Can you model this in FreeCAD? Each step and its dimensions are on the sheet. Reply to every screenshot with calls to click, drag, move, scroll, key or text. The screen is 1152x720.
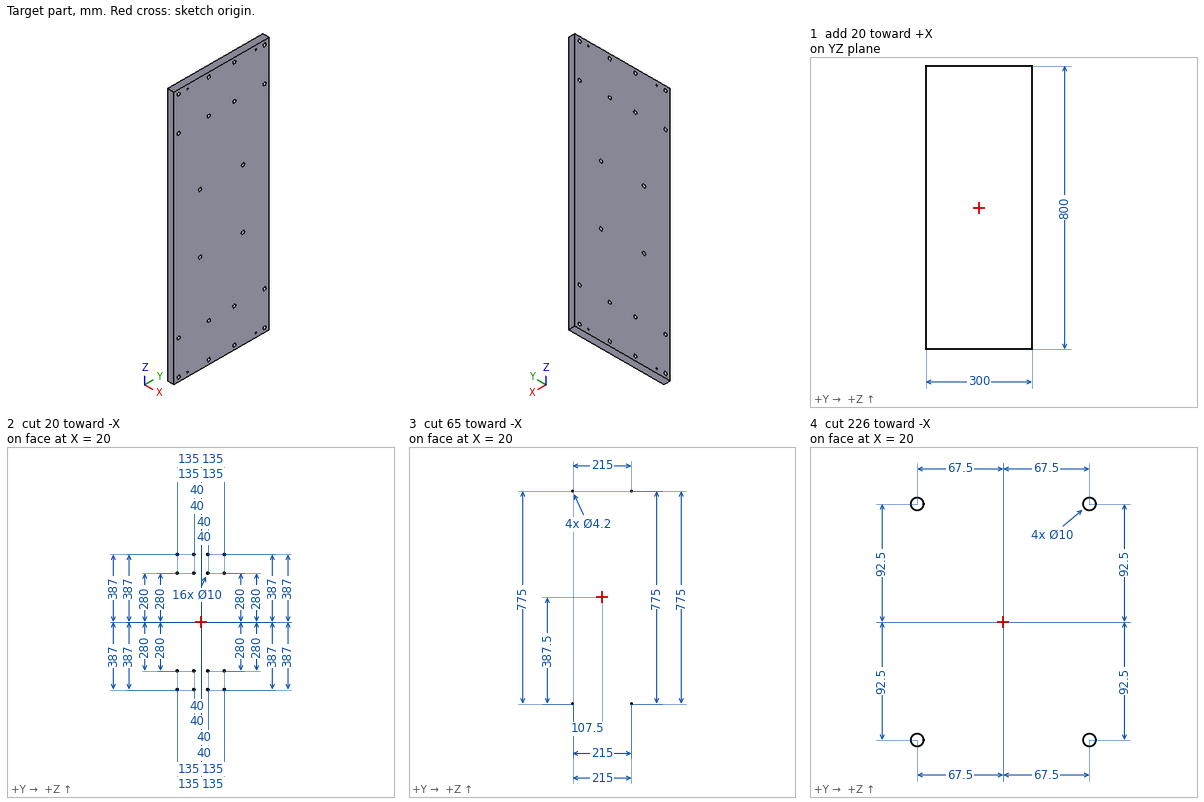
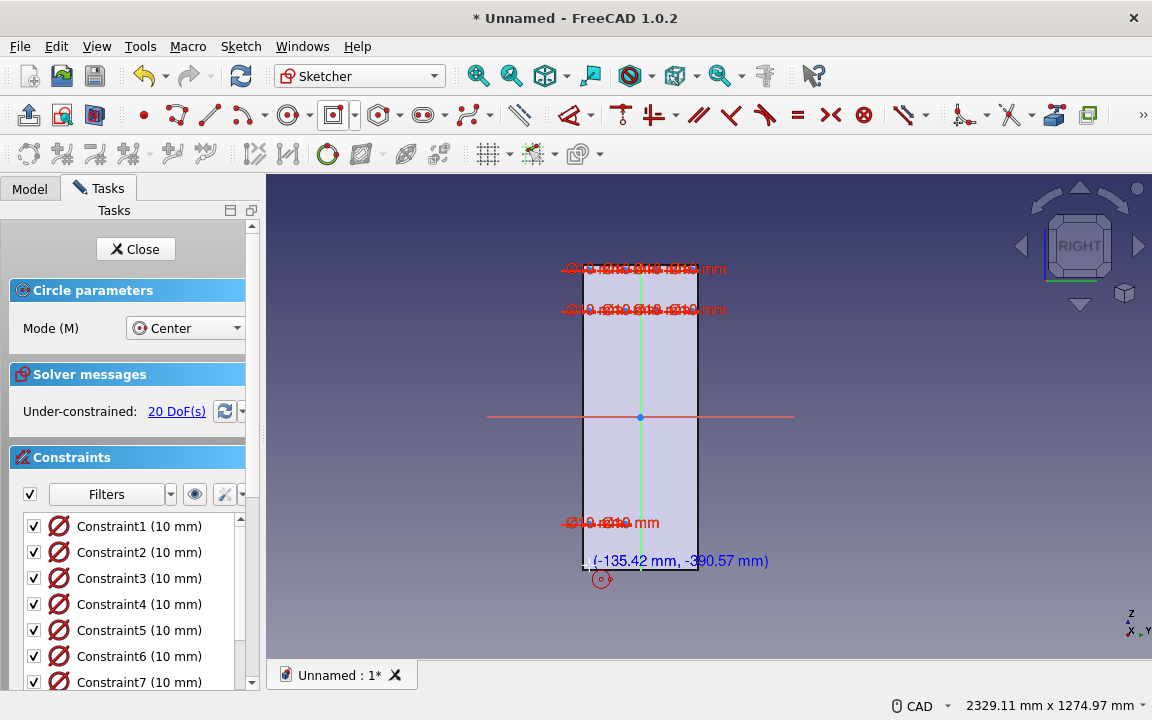
click(589, 565)
move(591, 563)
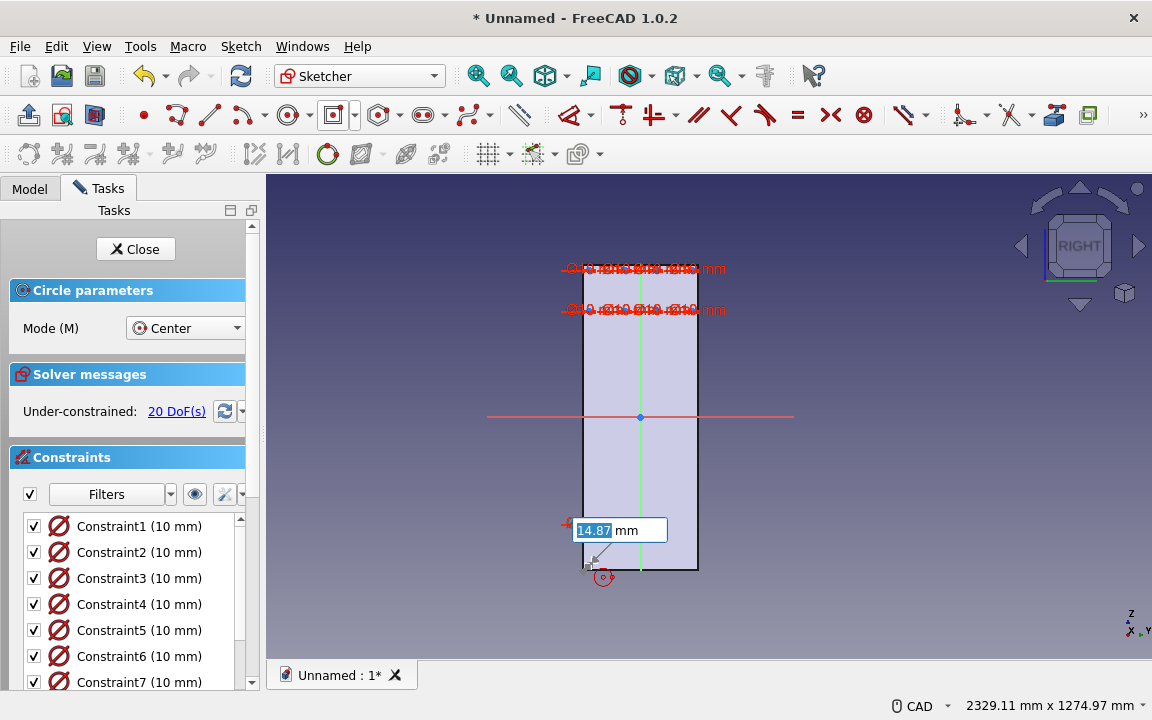
text(10)
key(Return)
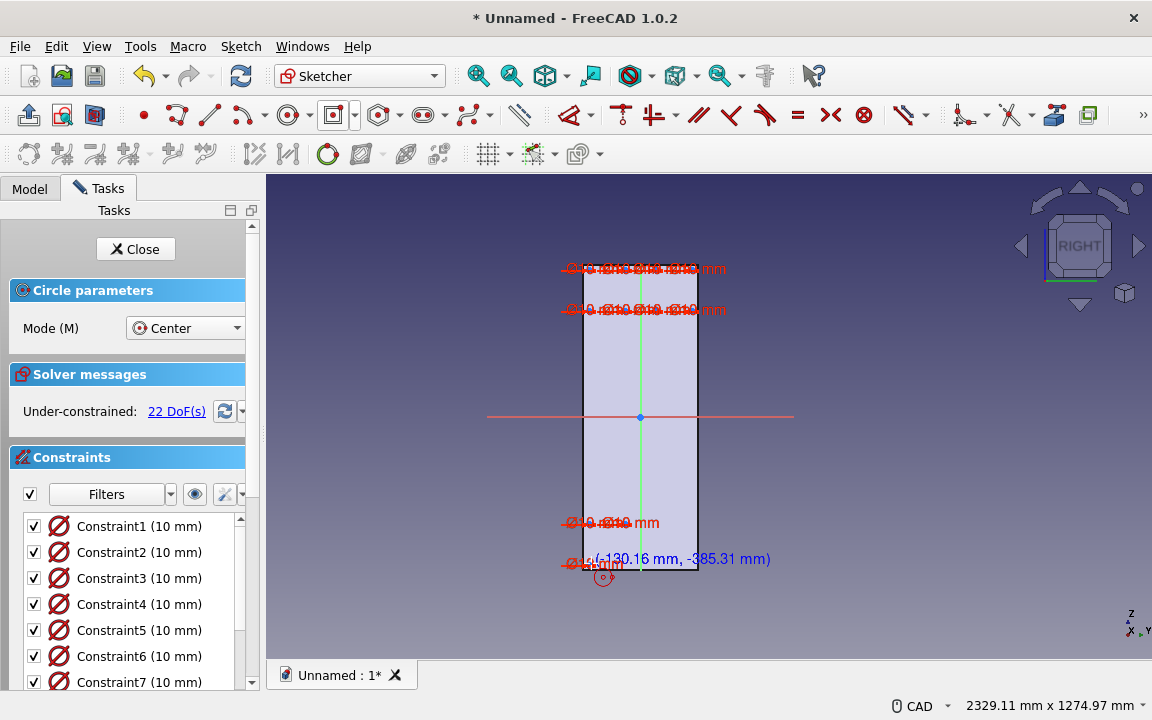
scroll(625, 565, up, 13)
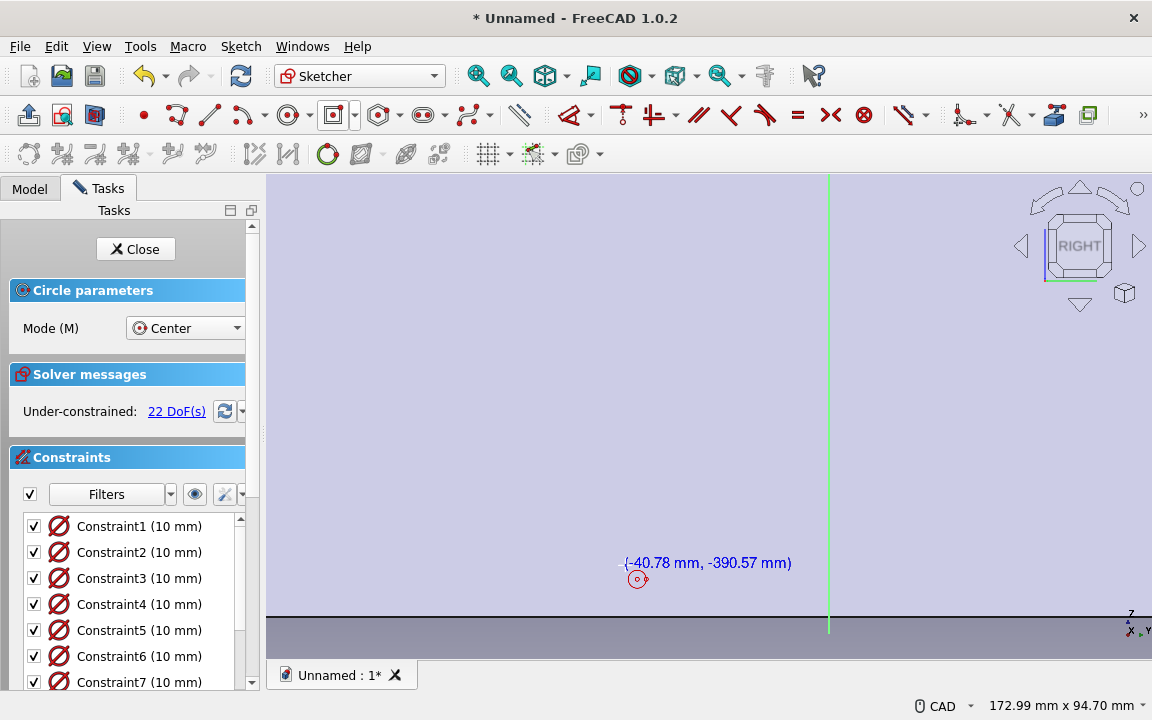
scroll(625, 565, down, 13)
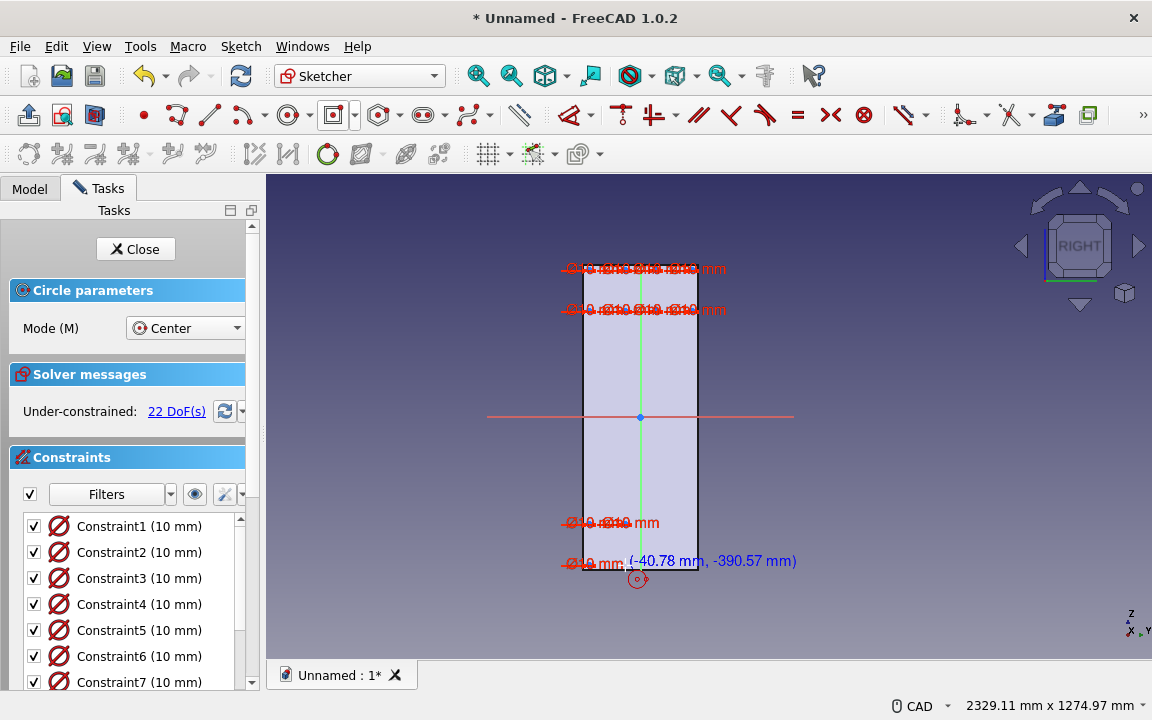
click(625, 565)
move(624, 563)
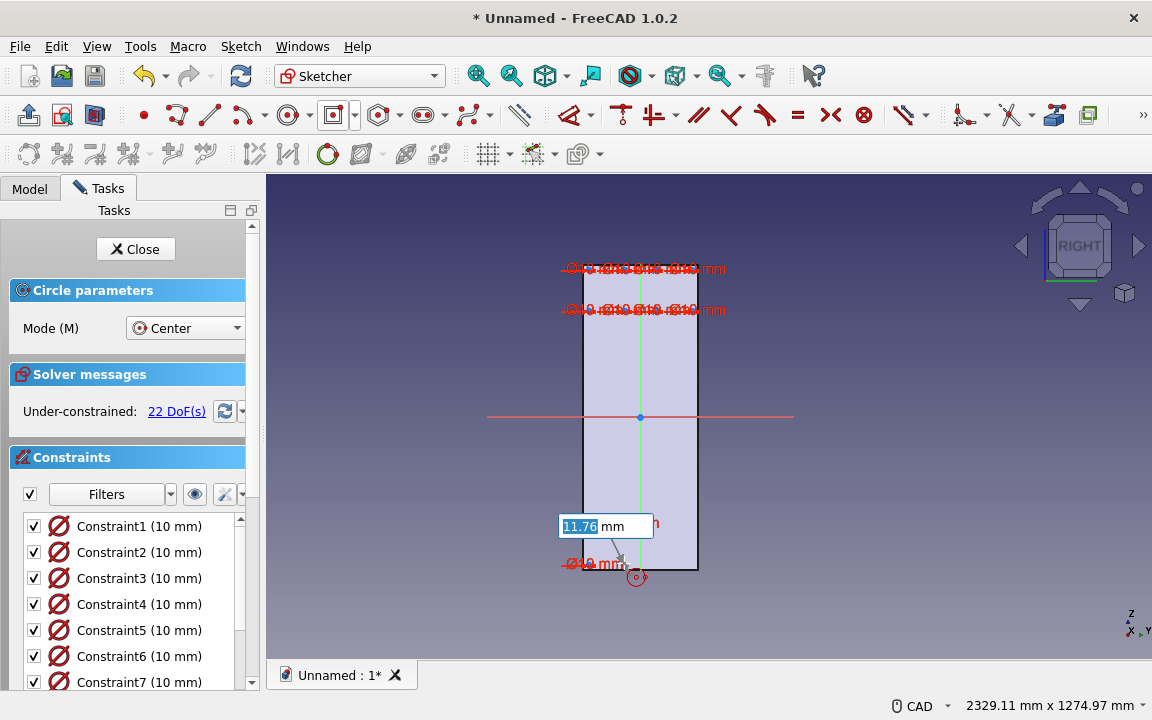
text(10)
key(Return)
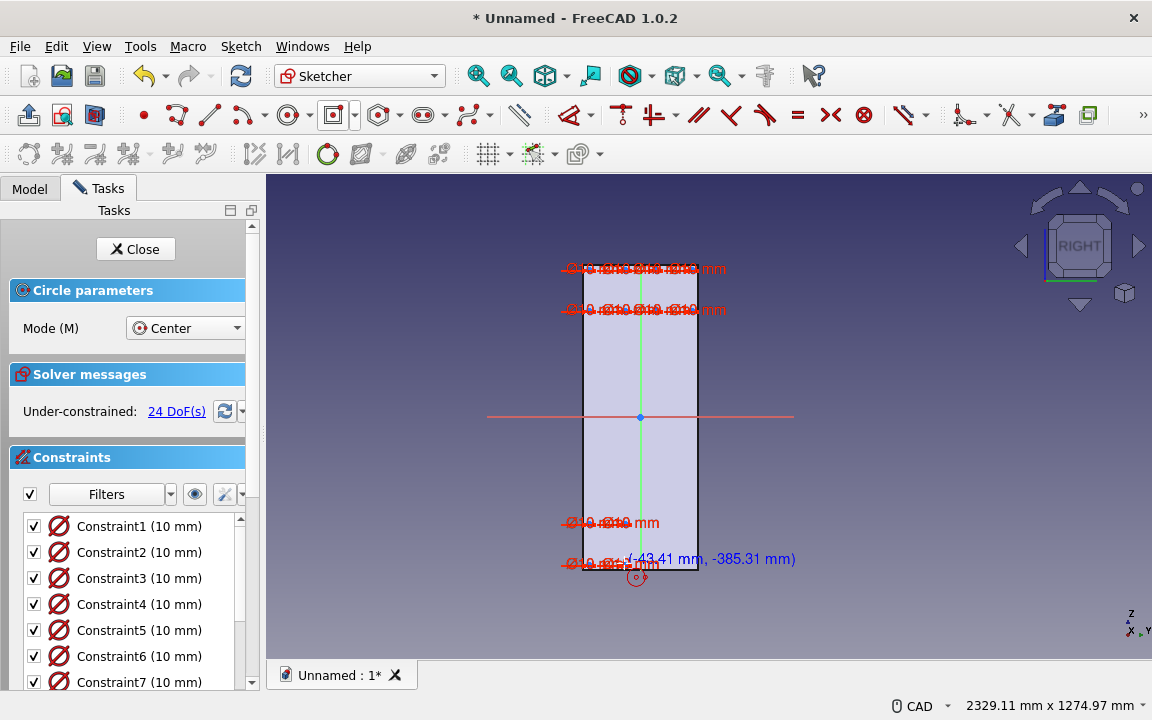
scroll(692, 524, up, 13)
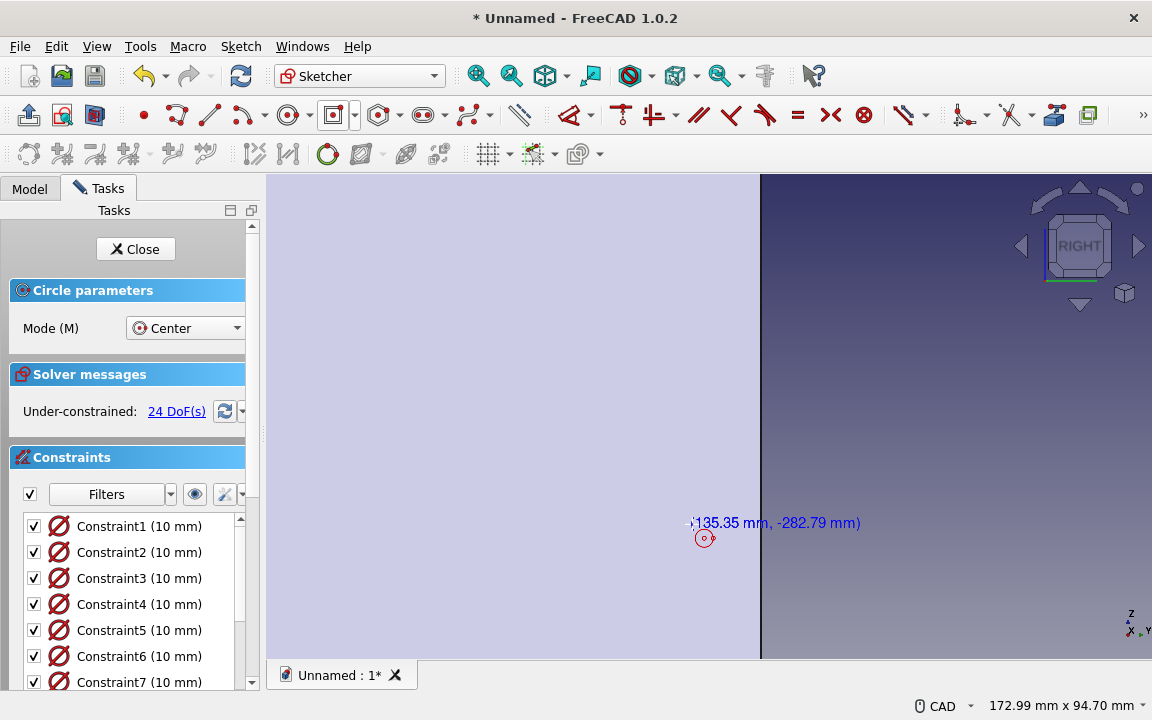
scroll(692, 524, down, 13)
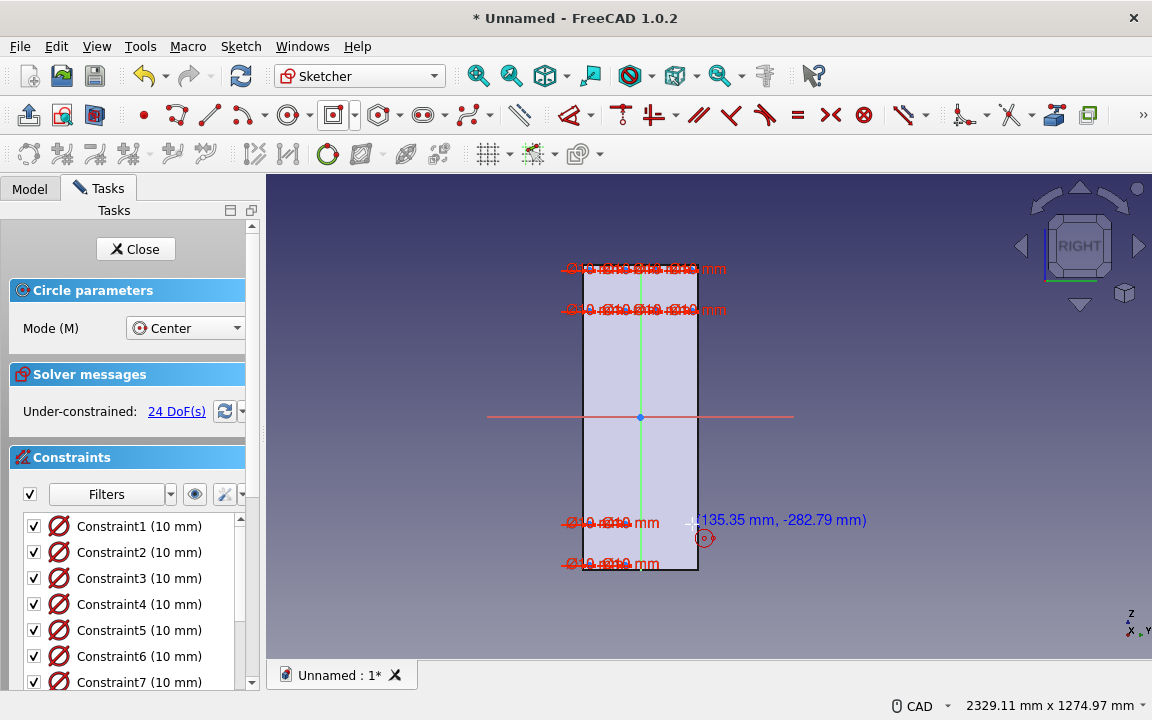
click(692, 524)
move(693, 523)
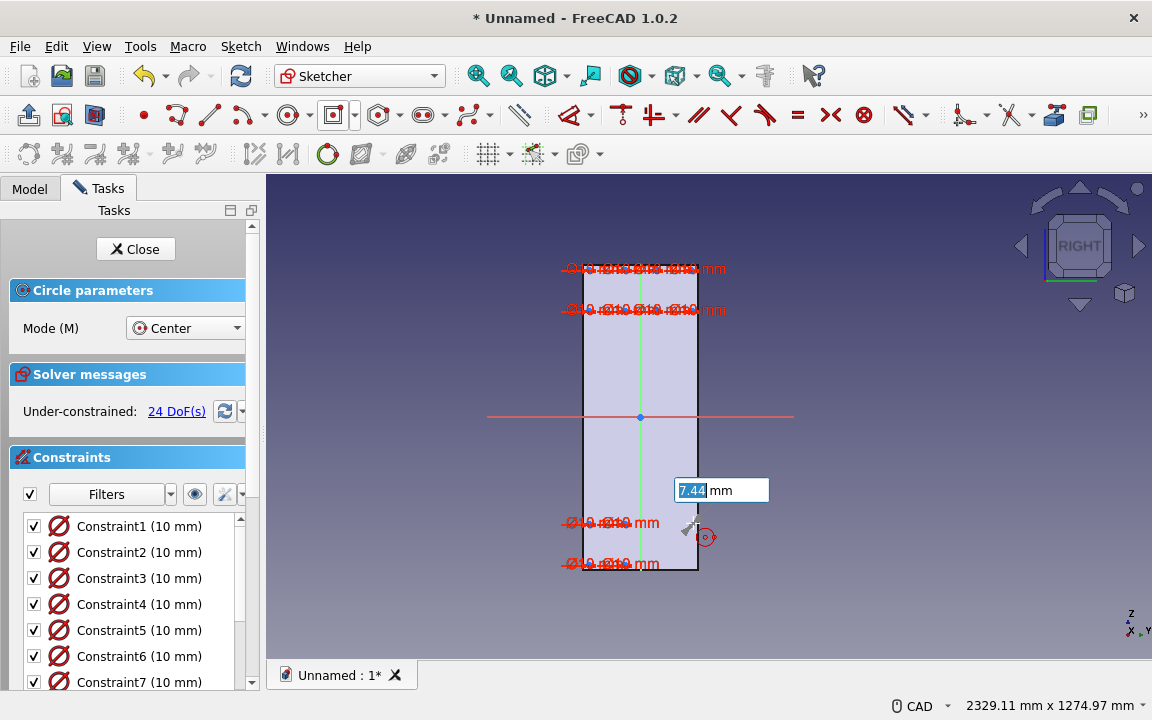
text(10)
key(Return)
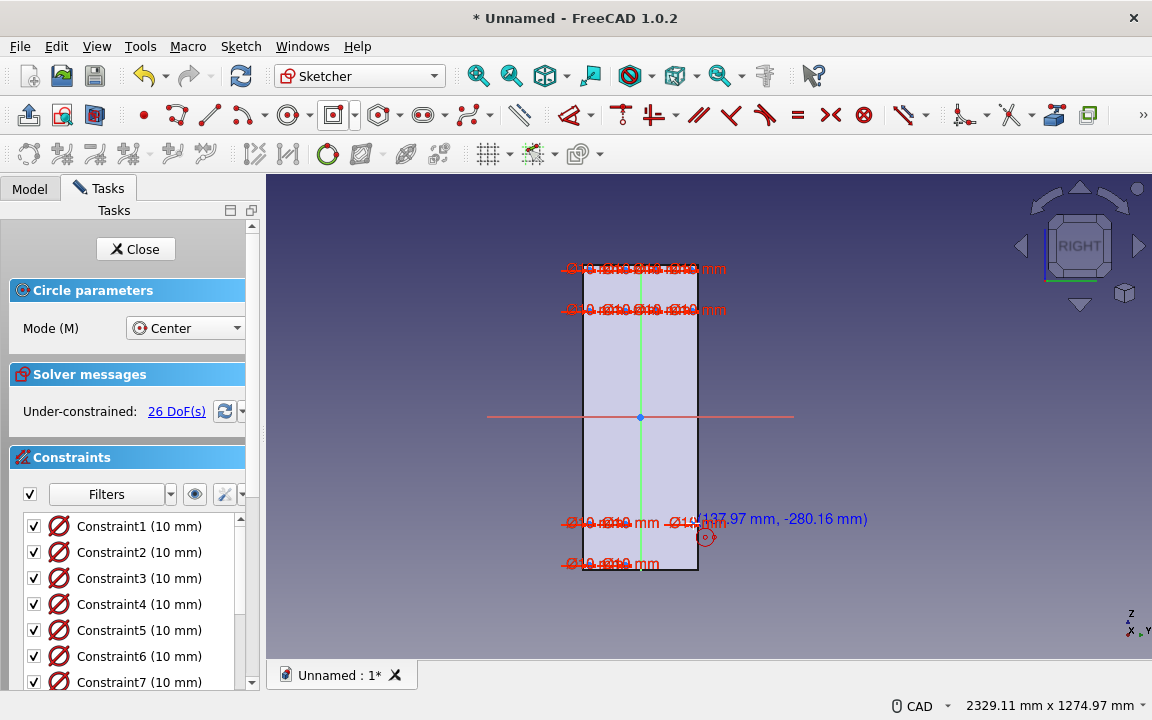
scroll(692, 565, up, 13)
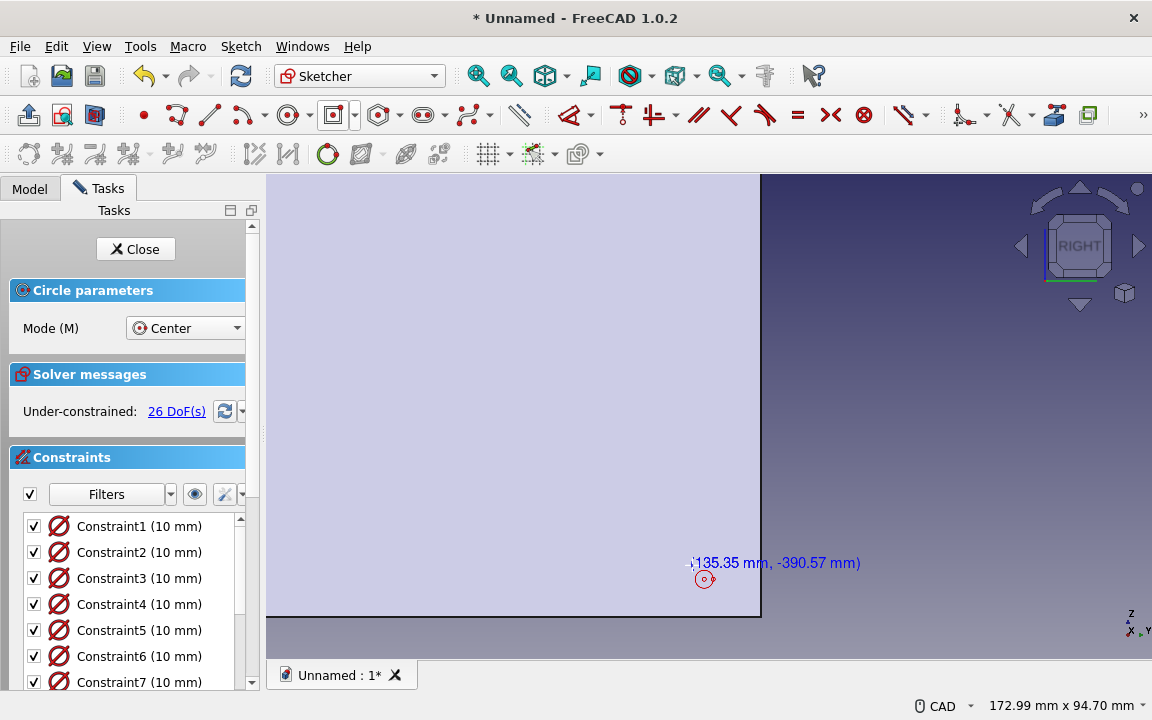
scroll(692, 565, down, 13)